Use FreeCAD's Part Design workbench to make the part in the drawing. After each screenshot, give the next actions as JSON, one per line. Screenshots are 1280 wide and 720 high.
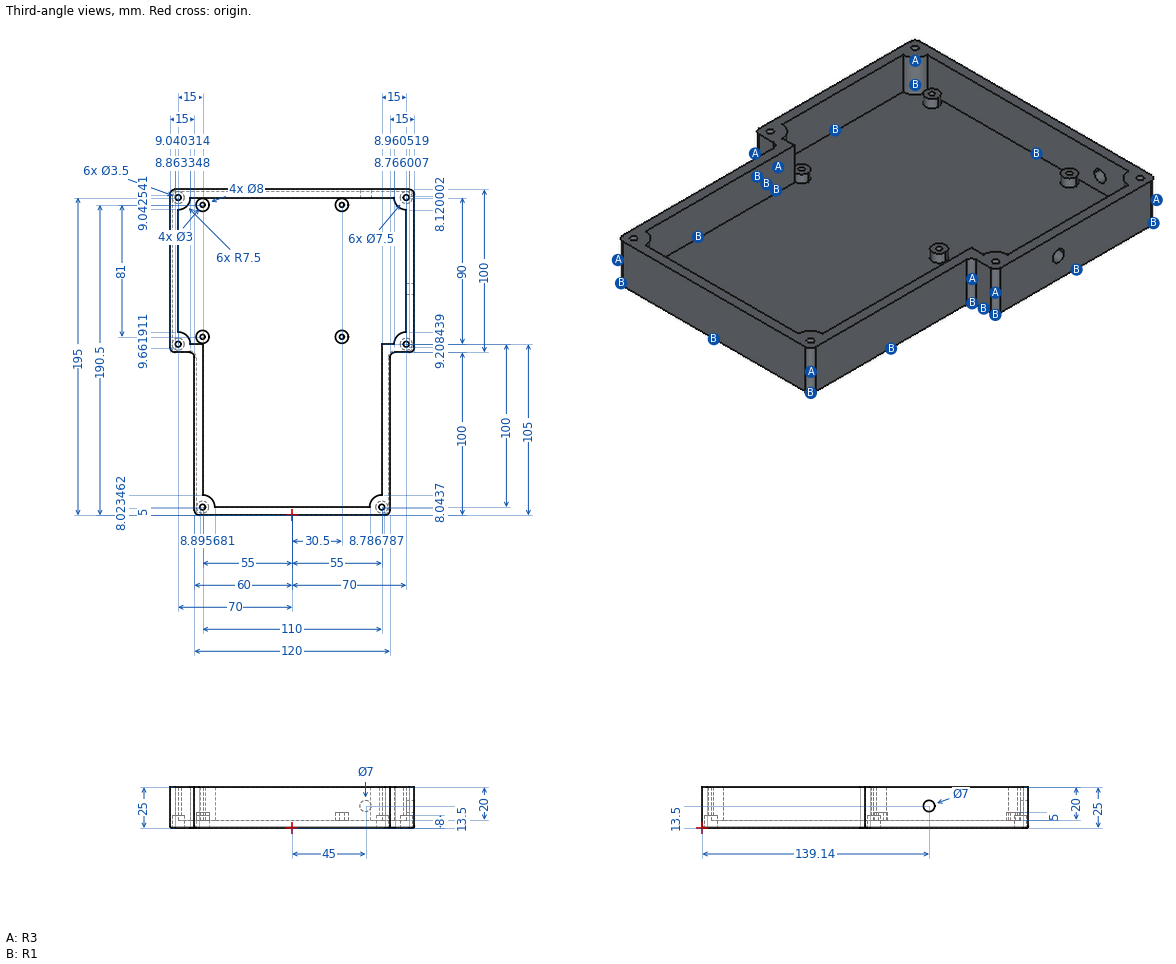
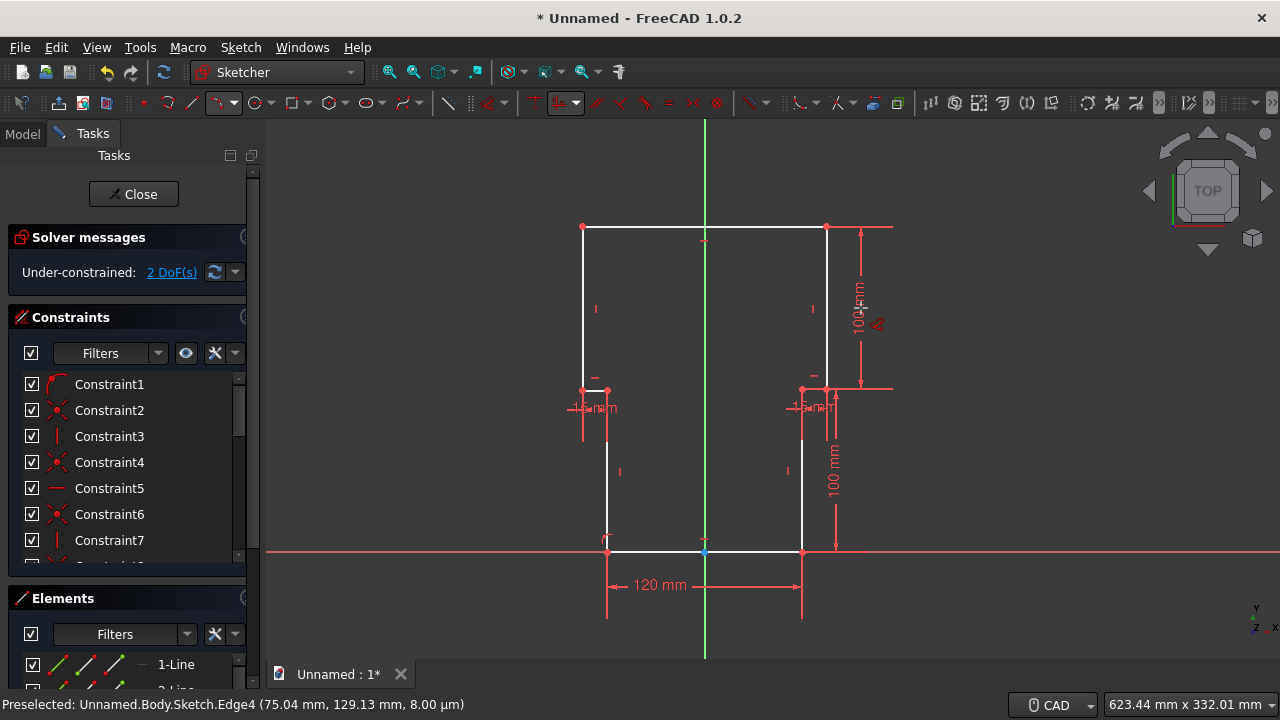
{"action": "left_click", "coordinate": [583, 276]}
{"action": "left_click", "coordinate": [549, 309]}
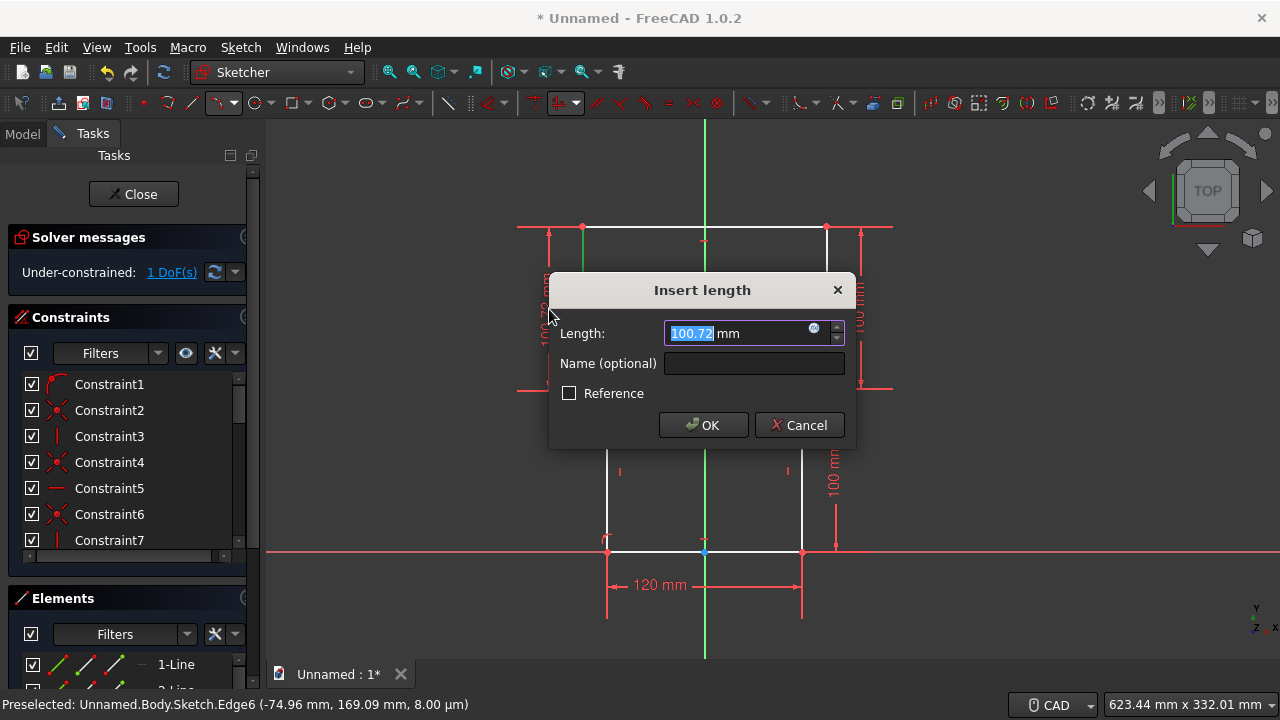
{"action": "type", "text": "100"}
{"action": "key", "text": "Return"}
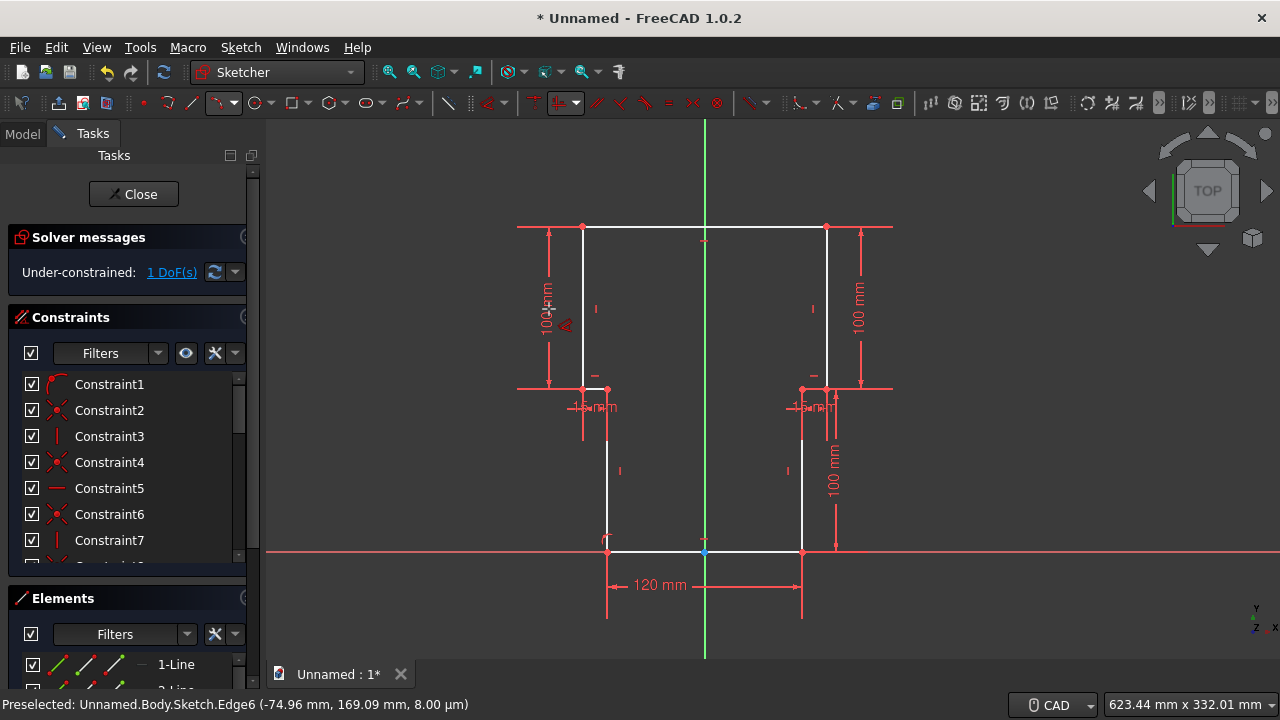
{"action": "left_click", "coordinate": [607, 552]}
{"action": "left_click", "coordinate": [656, 518]}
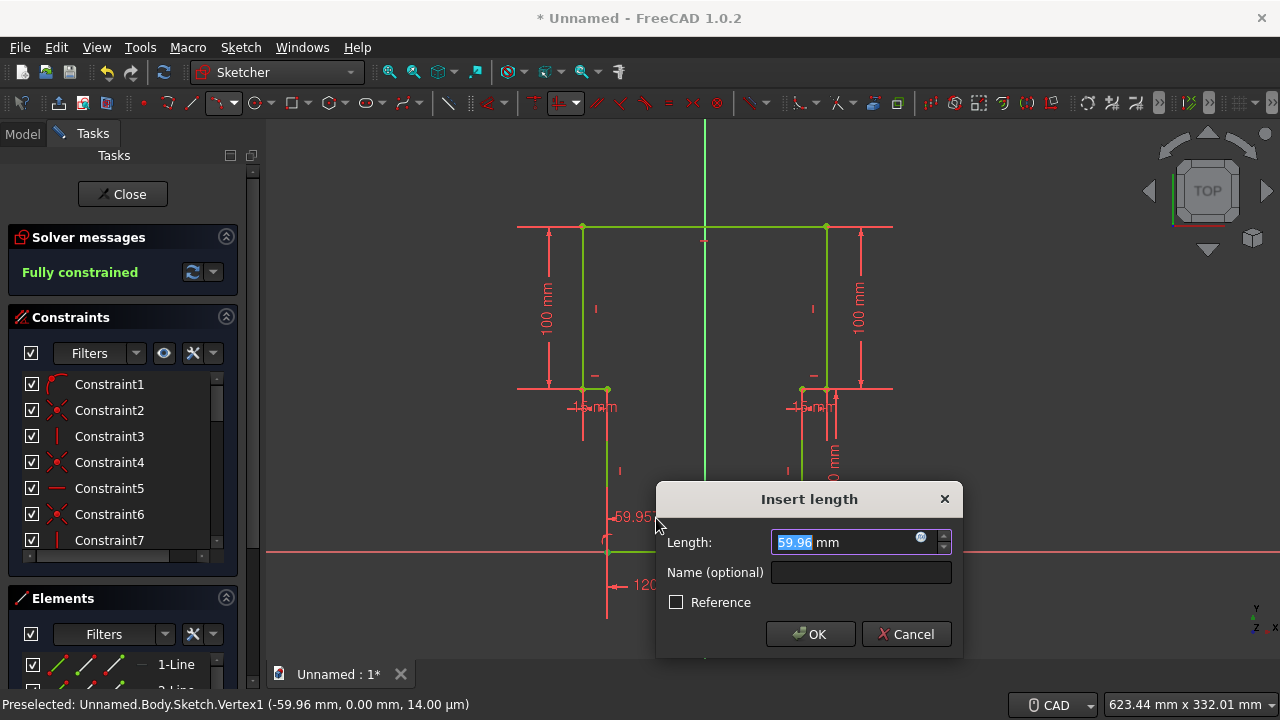
{"action": "type", "text": "60"}
{"action": "key", "text": "Return"}
{"action": "key", "text": "Escape"}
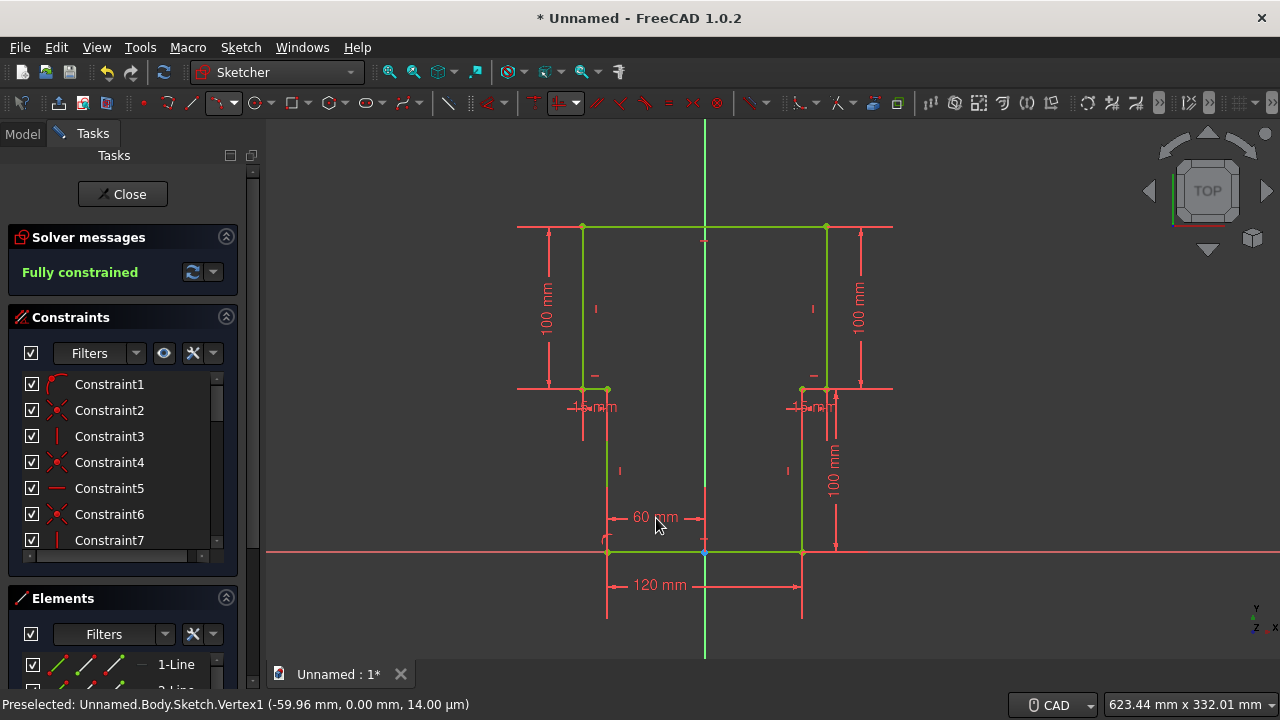
{"action": "left_click", "coordinate": [123, 194]}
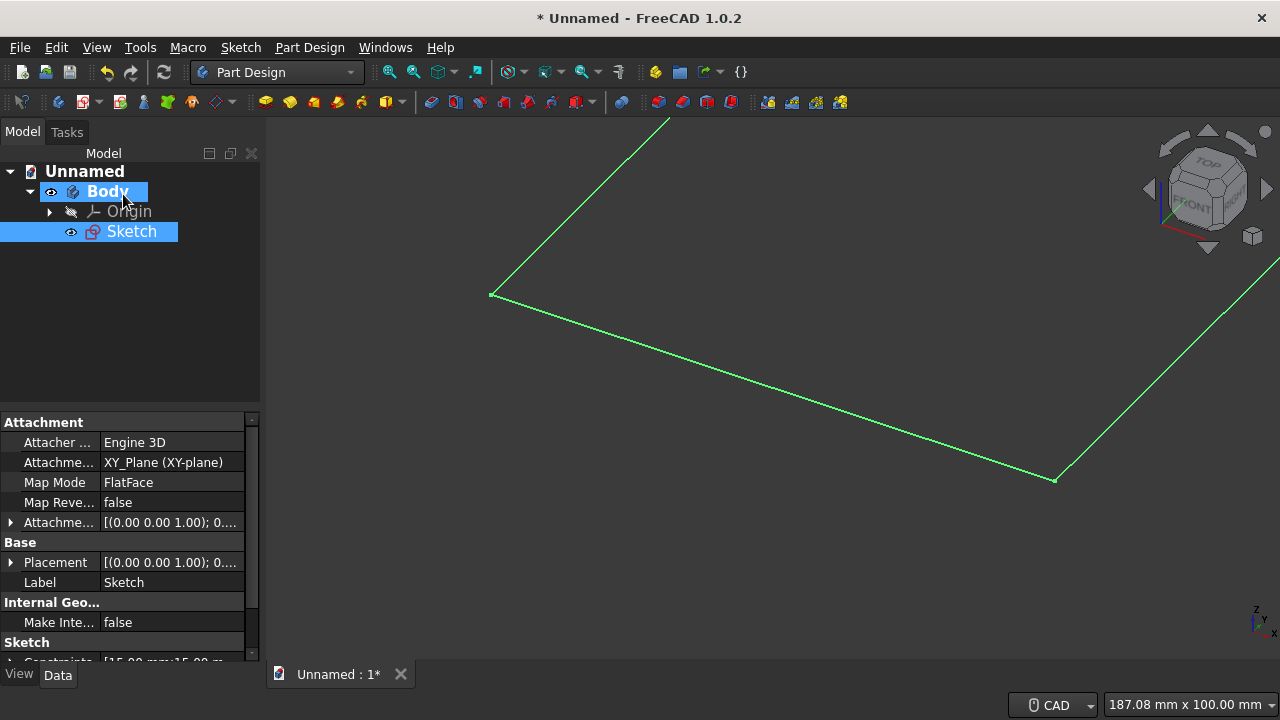
{"action": "left_click", "coordinate": [266, 102]}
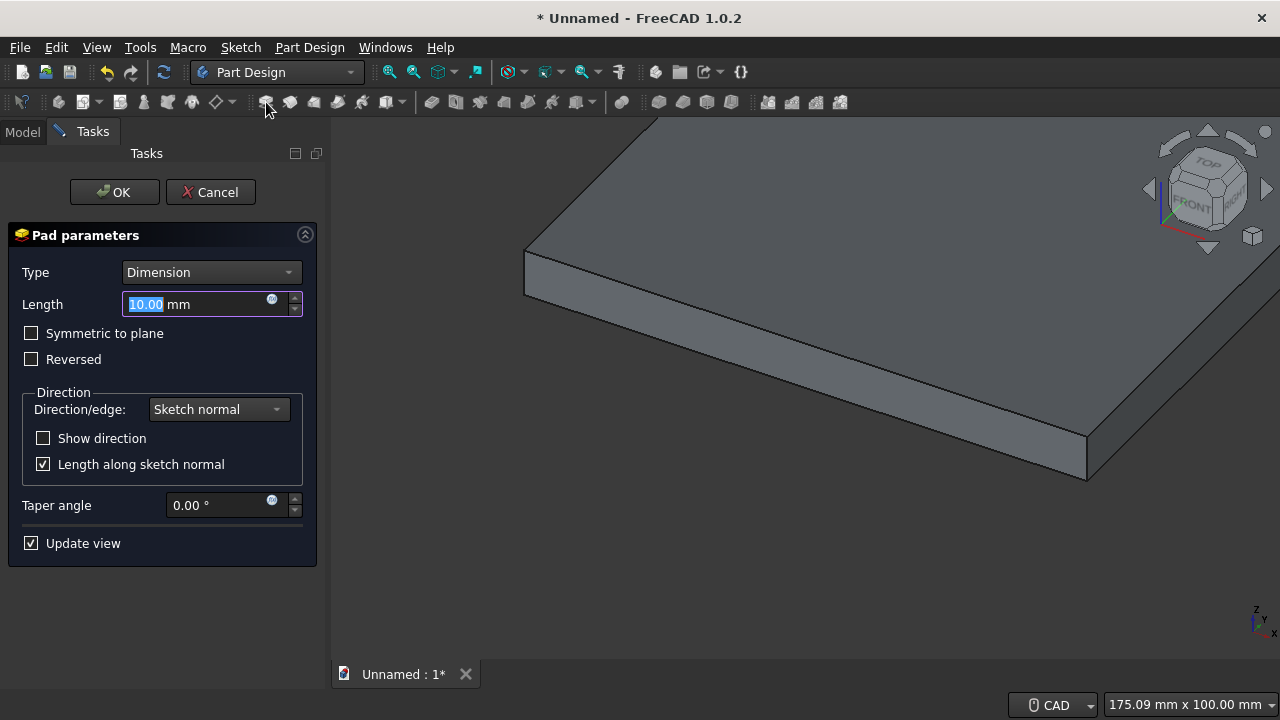
{"action": "type", "text": "25"}
{"action": "key", "text": "Tab"}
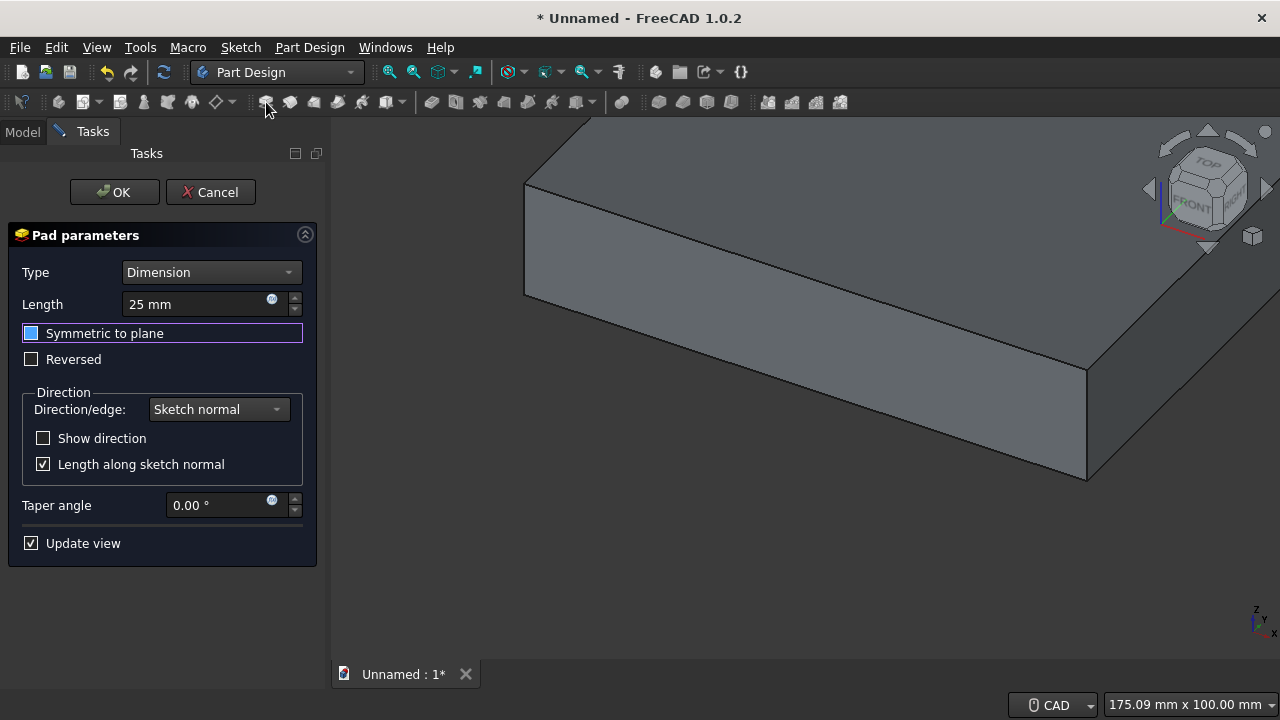
{"action": "left_click", "coordinate": [115, 192]}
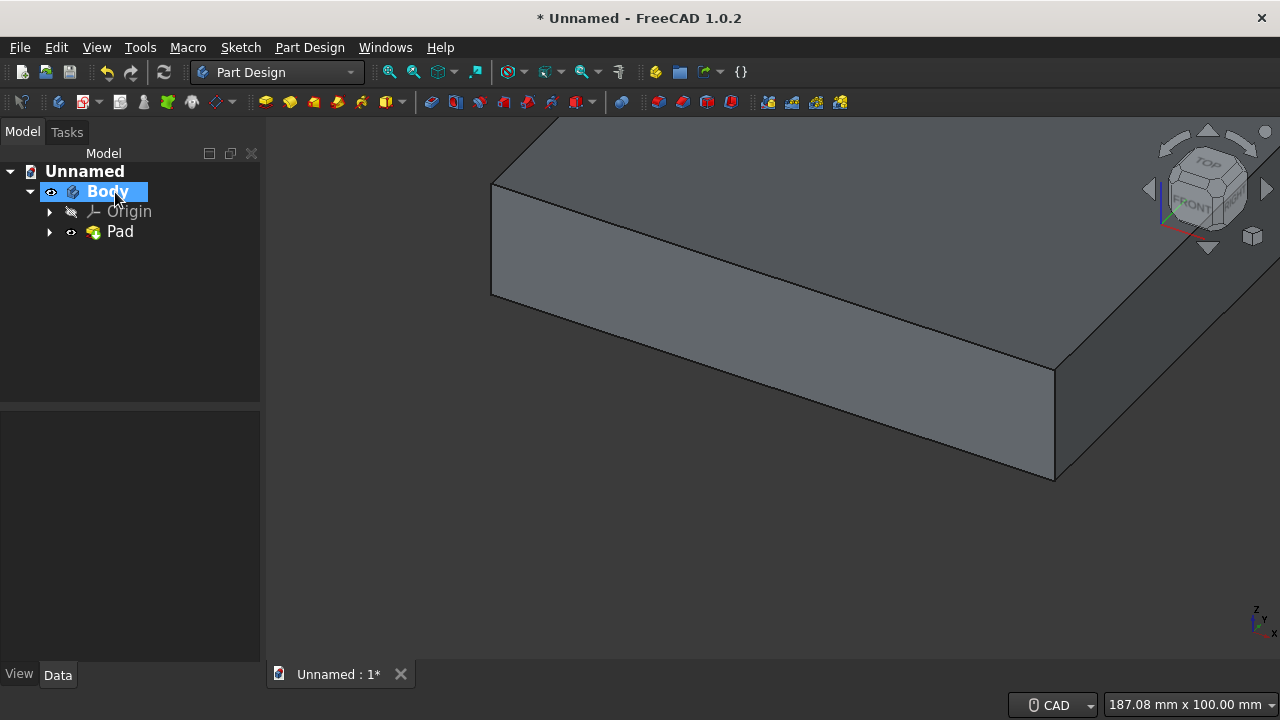
{"action": "key", "text": "v f"}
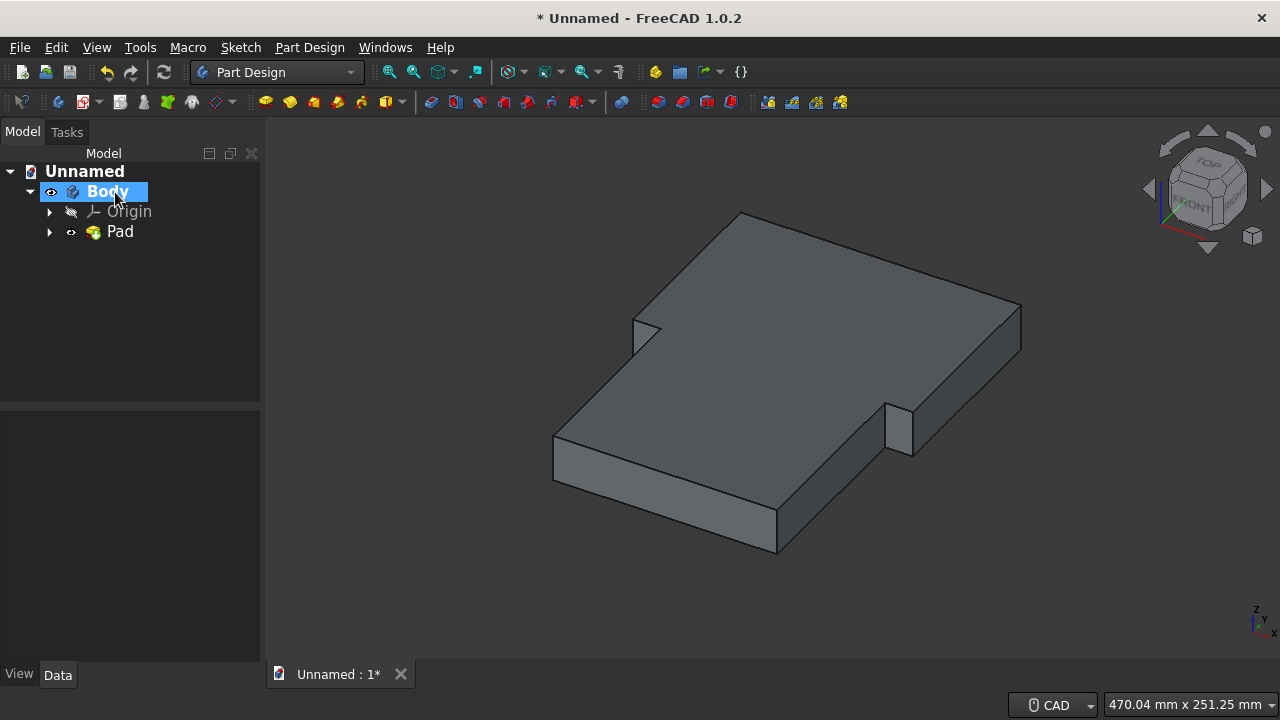
{"action": "left_click", "coordinate": [804, 334]}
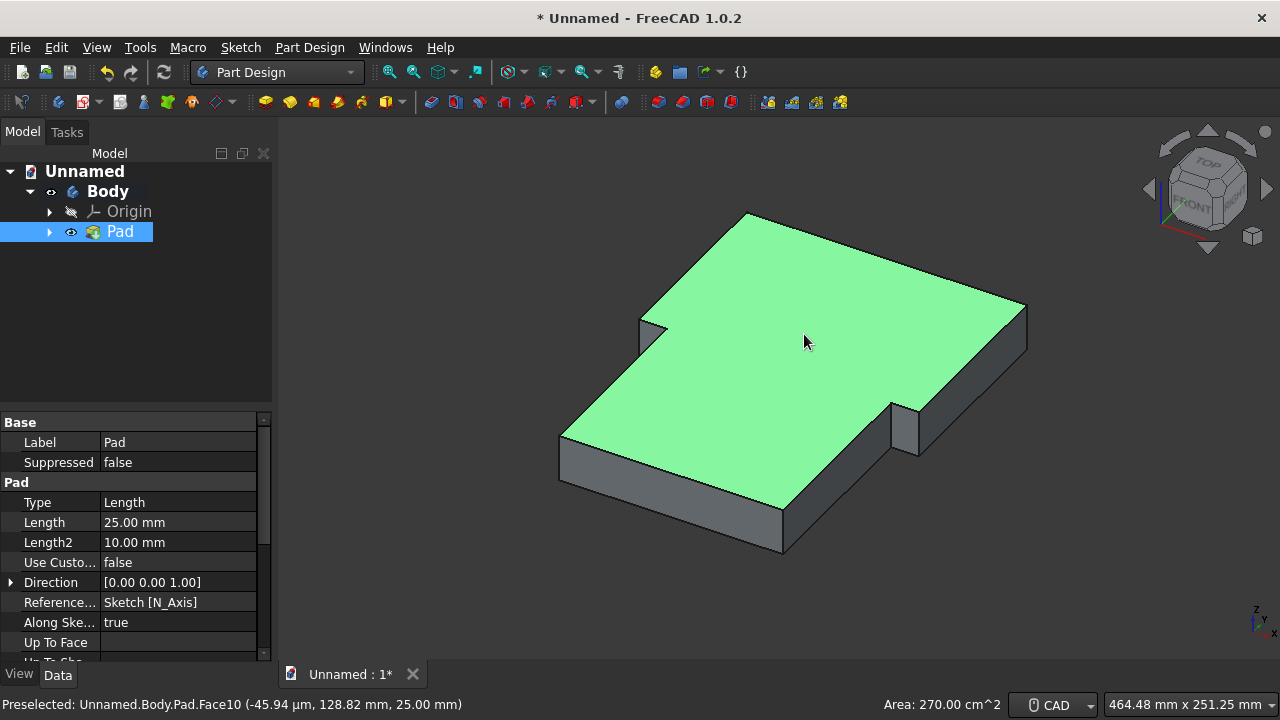
{"action": "left_click", "coordinate": [84, 102]}